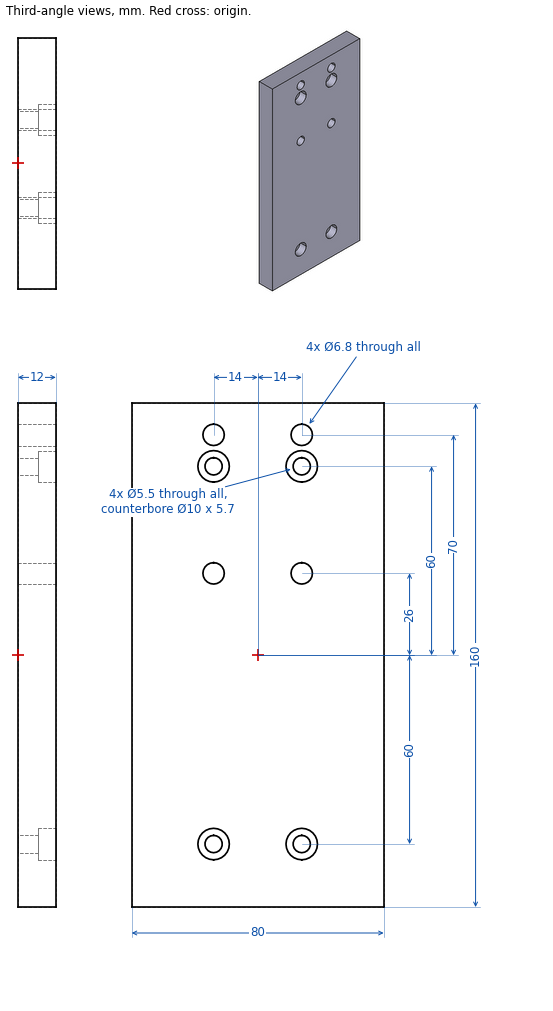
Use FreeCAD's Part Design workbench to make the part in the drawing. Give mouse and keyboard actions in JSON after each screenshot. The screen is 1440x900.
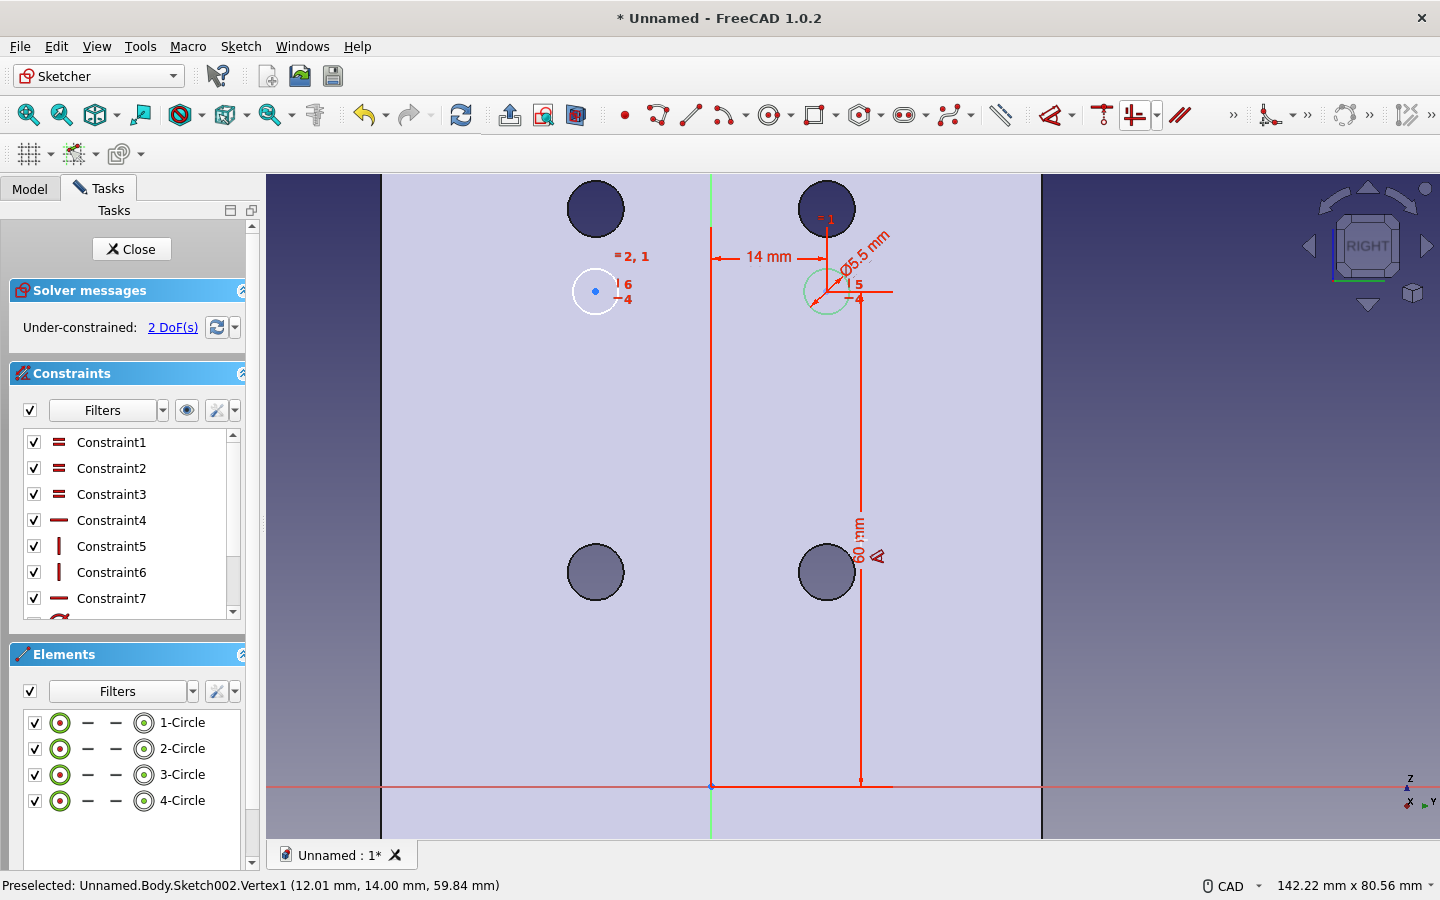
{"action": "left_click", "coordinate": [596, 292]}
{"action": "left_click", "coordinate": [654, 258]}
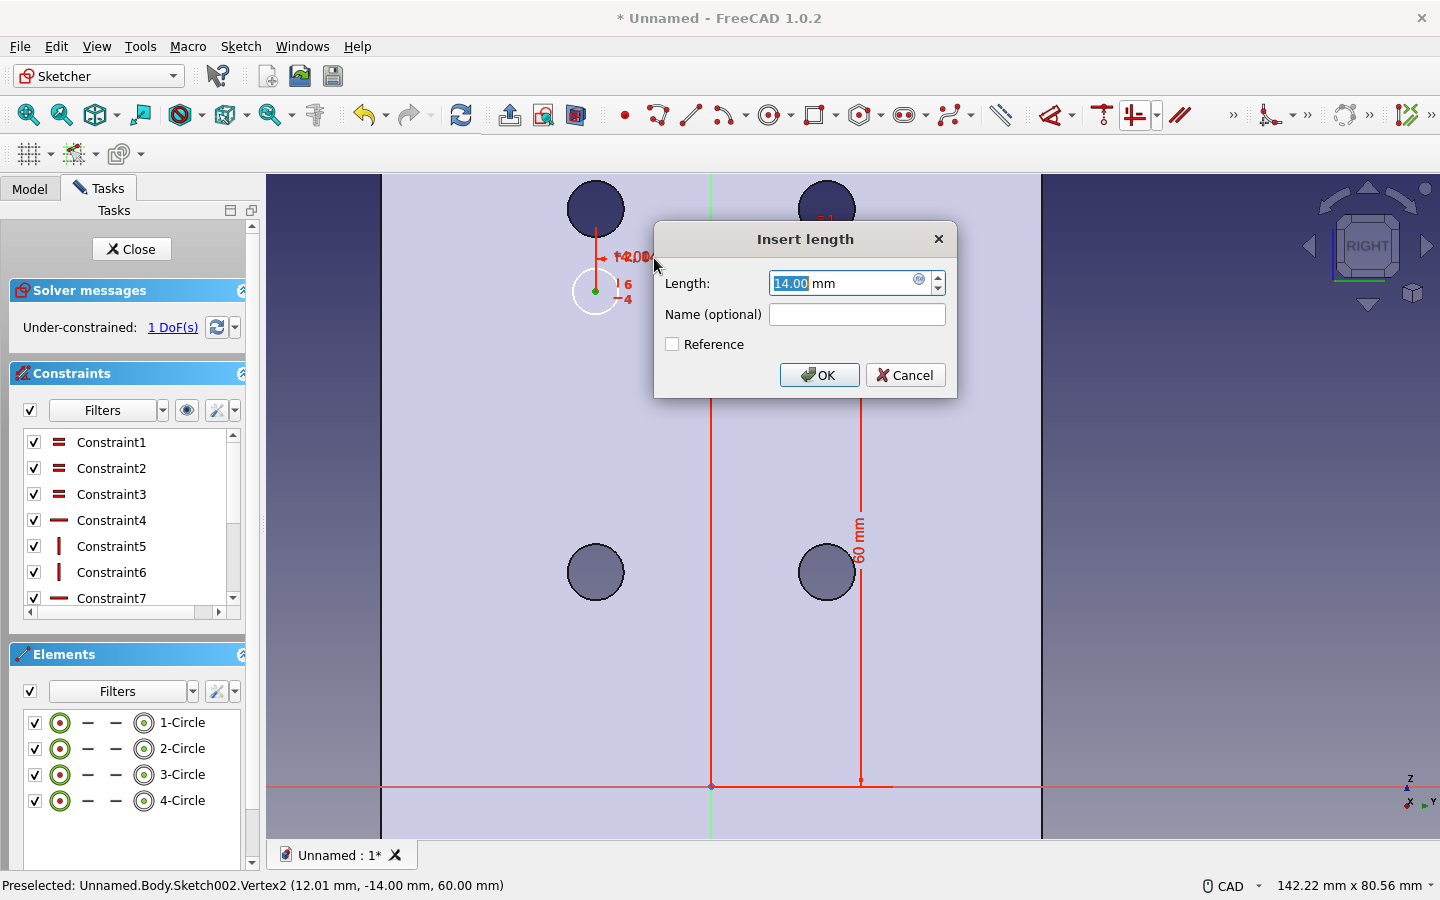
{"action": "type", "text": "14"}
{"action": "key", "text": "Return"}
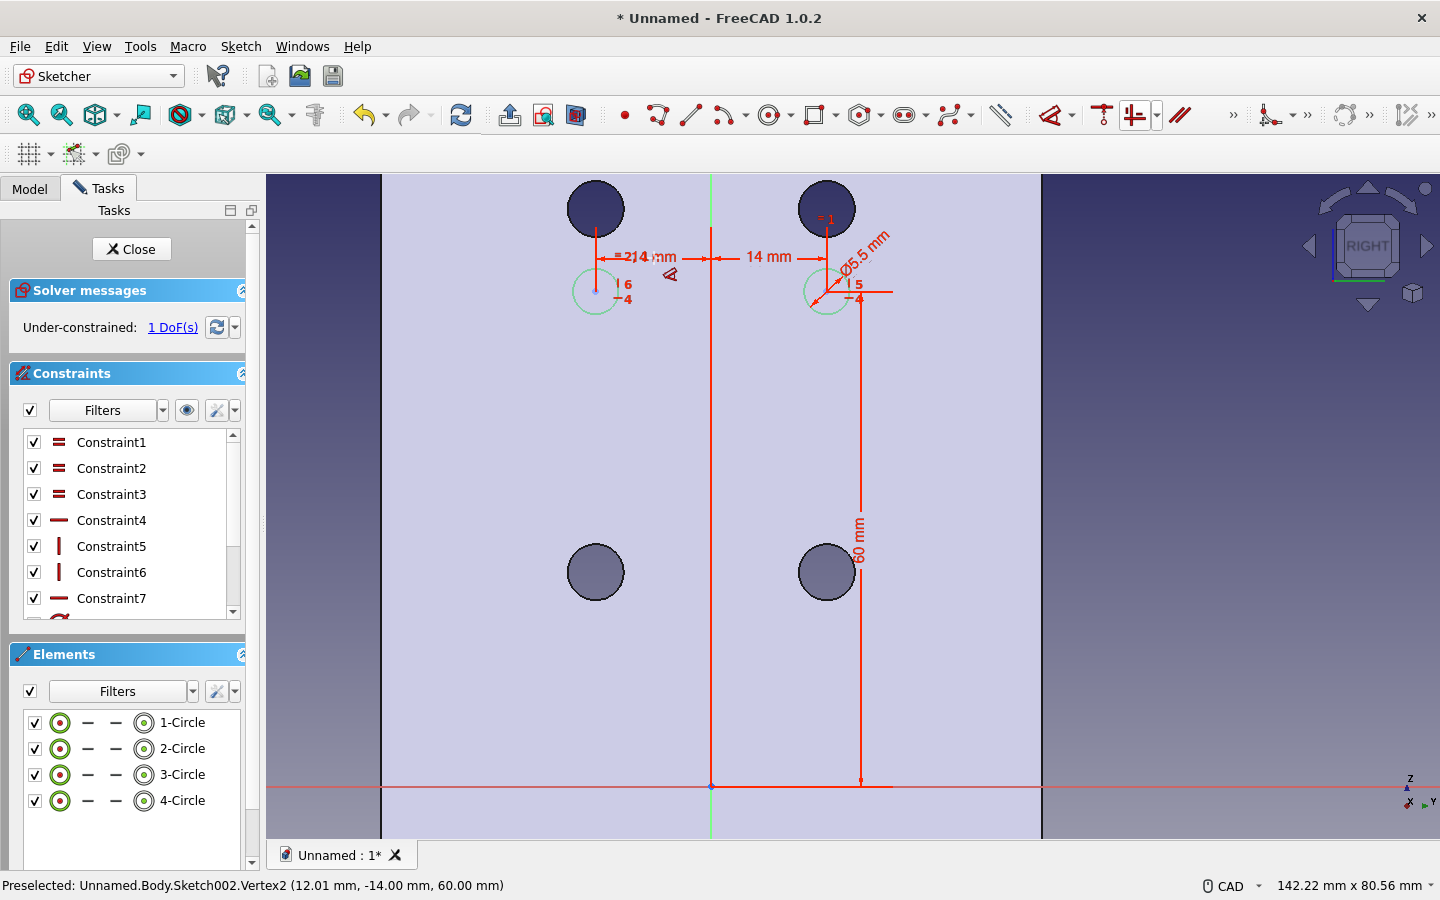
{"action": "scroll", "coordinate": [844, 278], "scroll_direction": "down", "scroll_amount": 4}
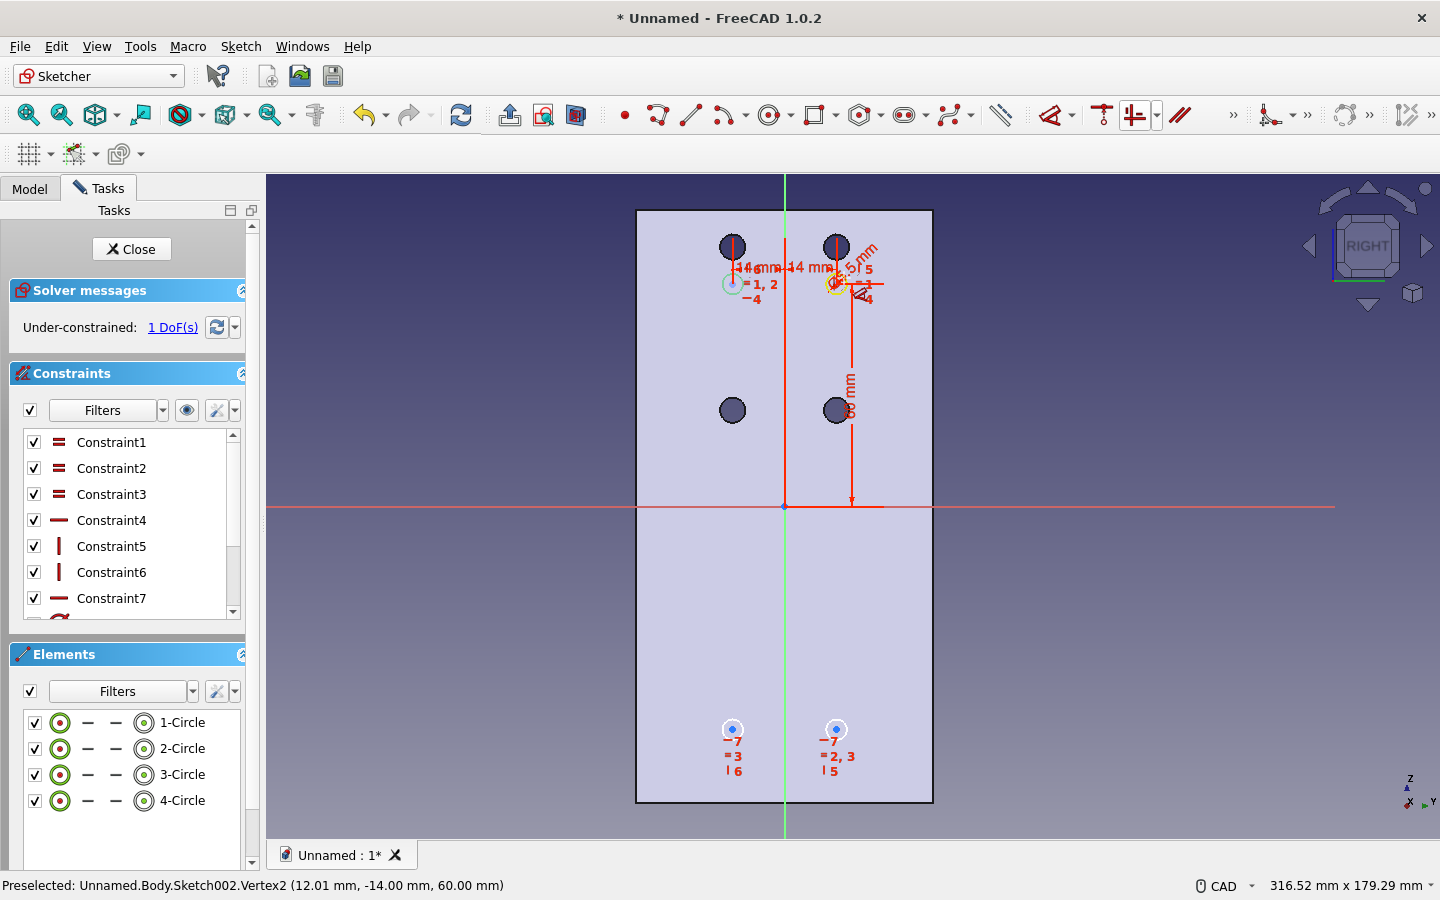
{"action": "left_click", "coordinate": [837, 730]}
{"action": "left_click", "coordinate": [871, 618]}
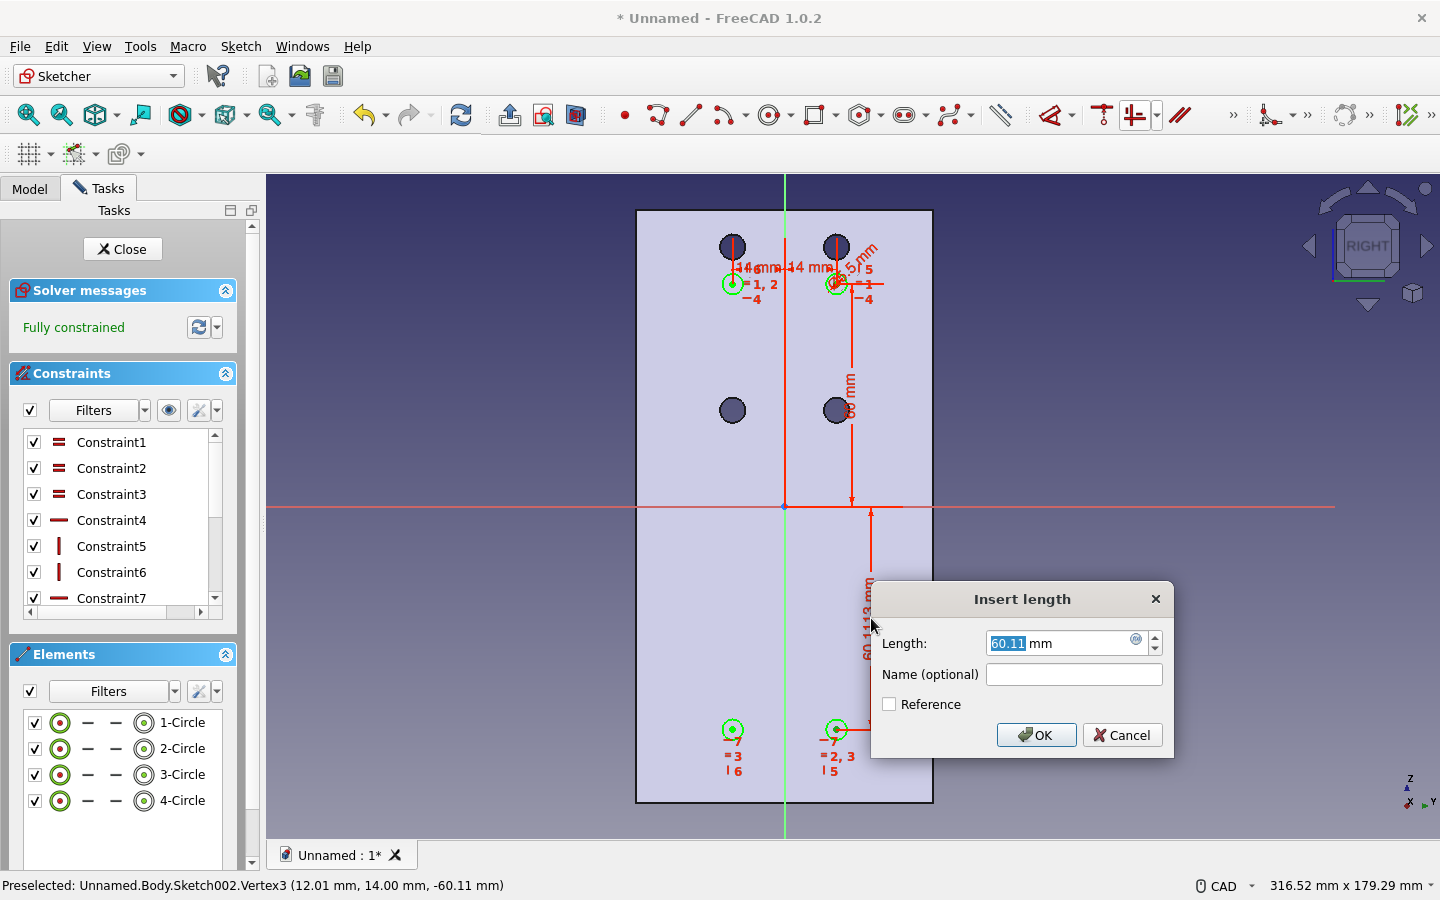
{"action": "type", "text": "60"}
{"action": "key", "text": "Return"}
{"action": "key", "text": "Escape"}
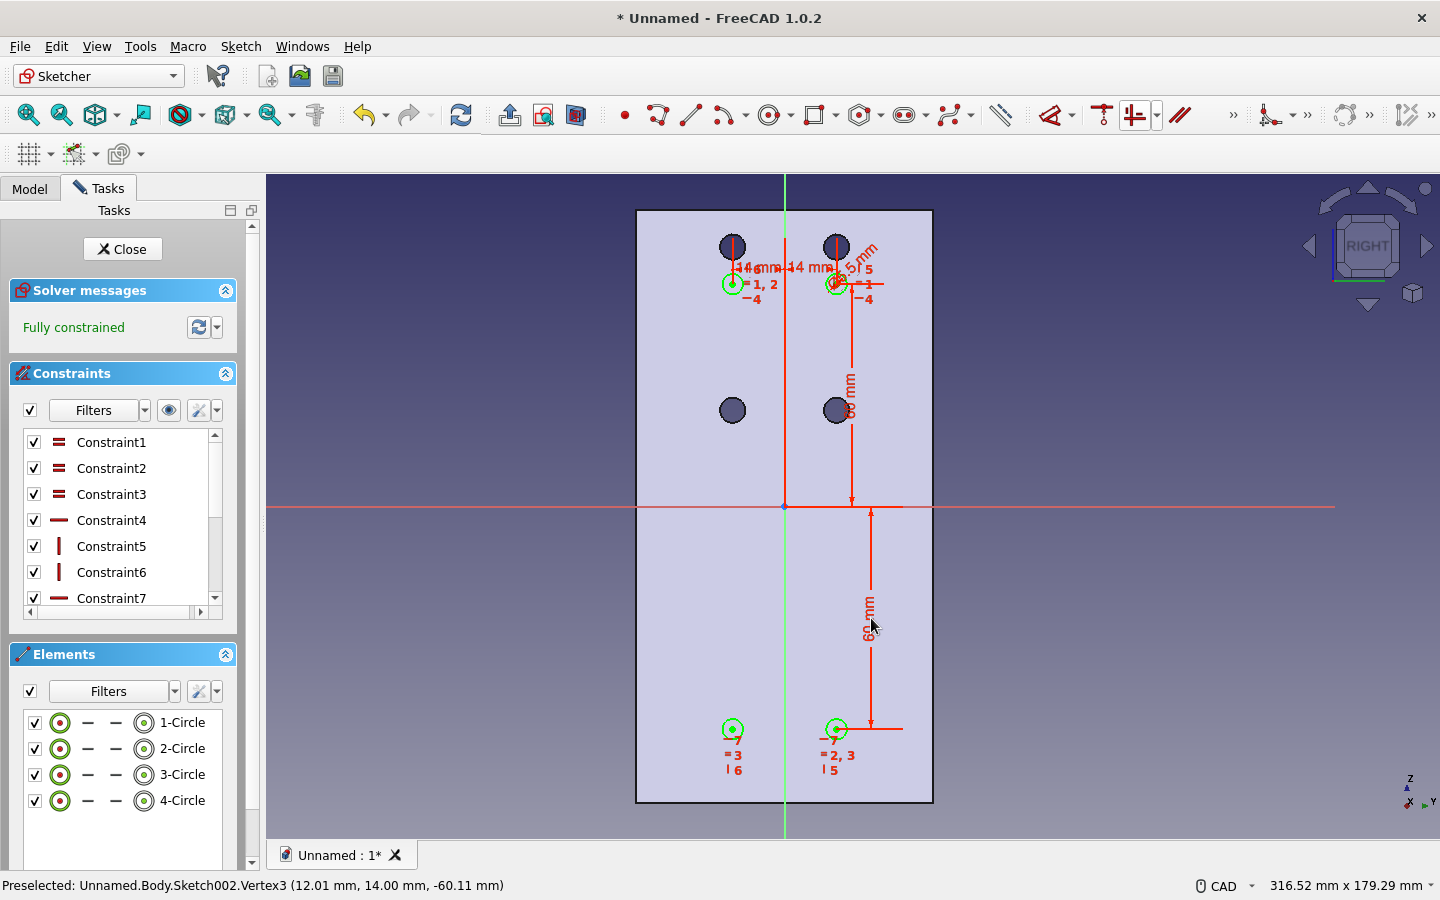
{"action": "left_click", "coordinate": [123, 249]}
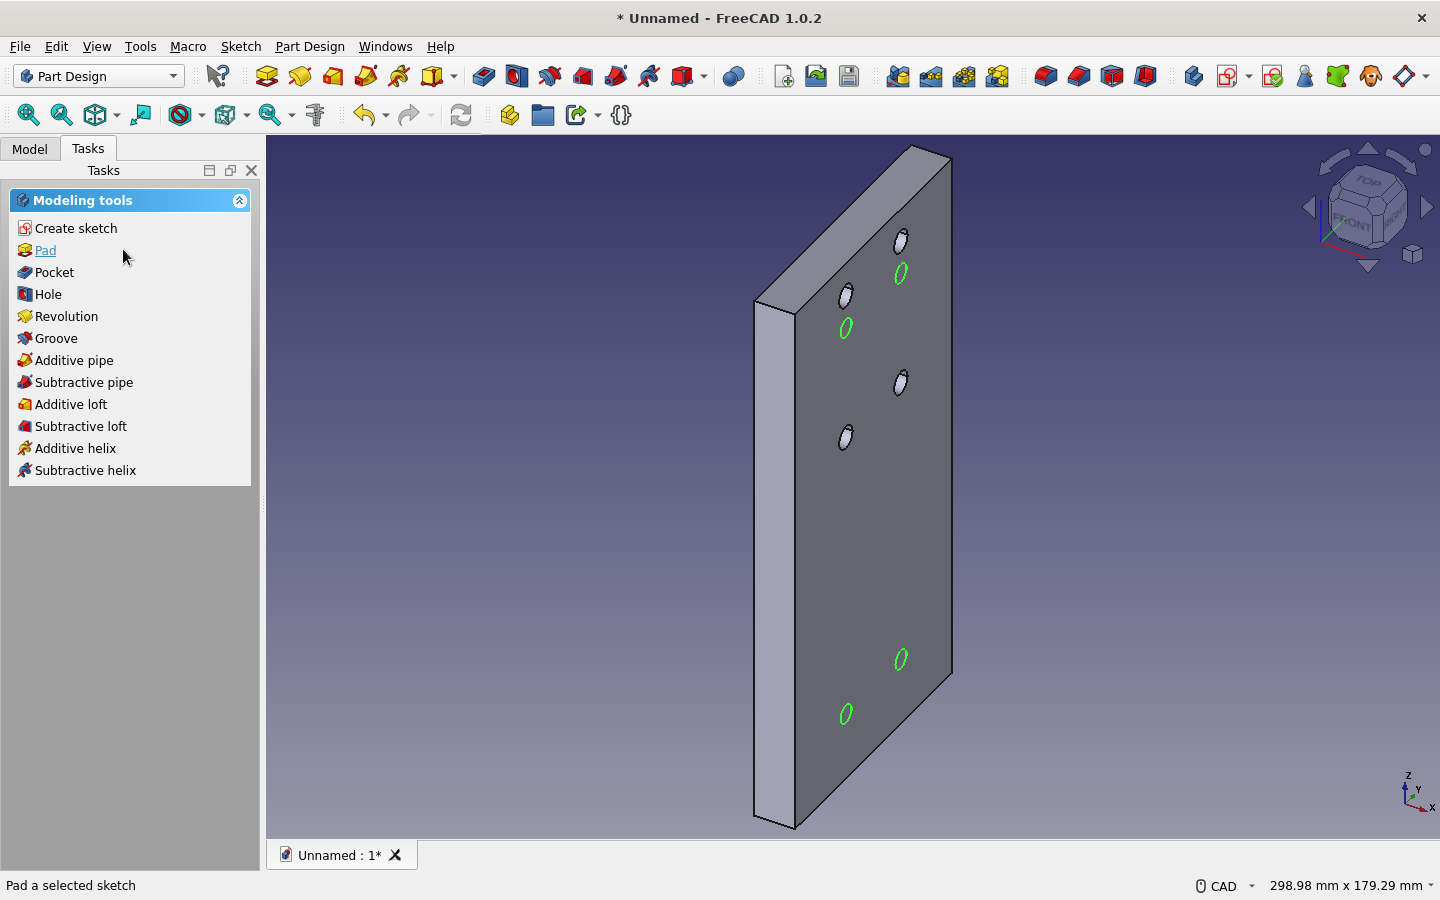
{"action": "left_click", "coordinate": [517, 76]}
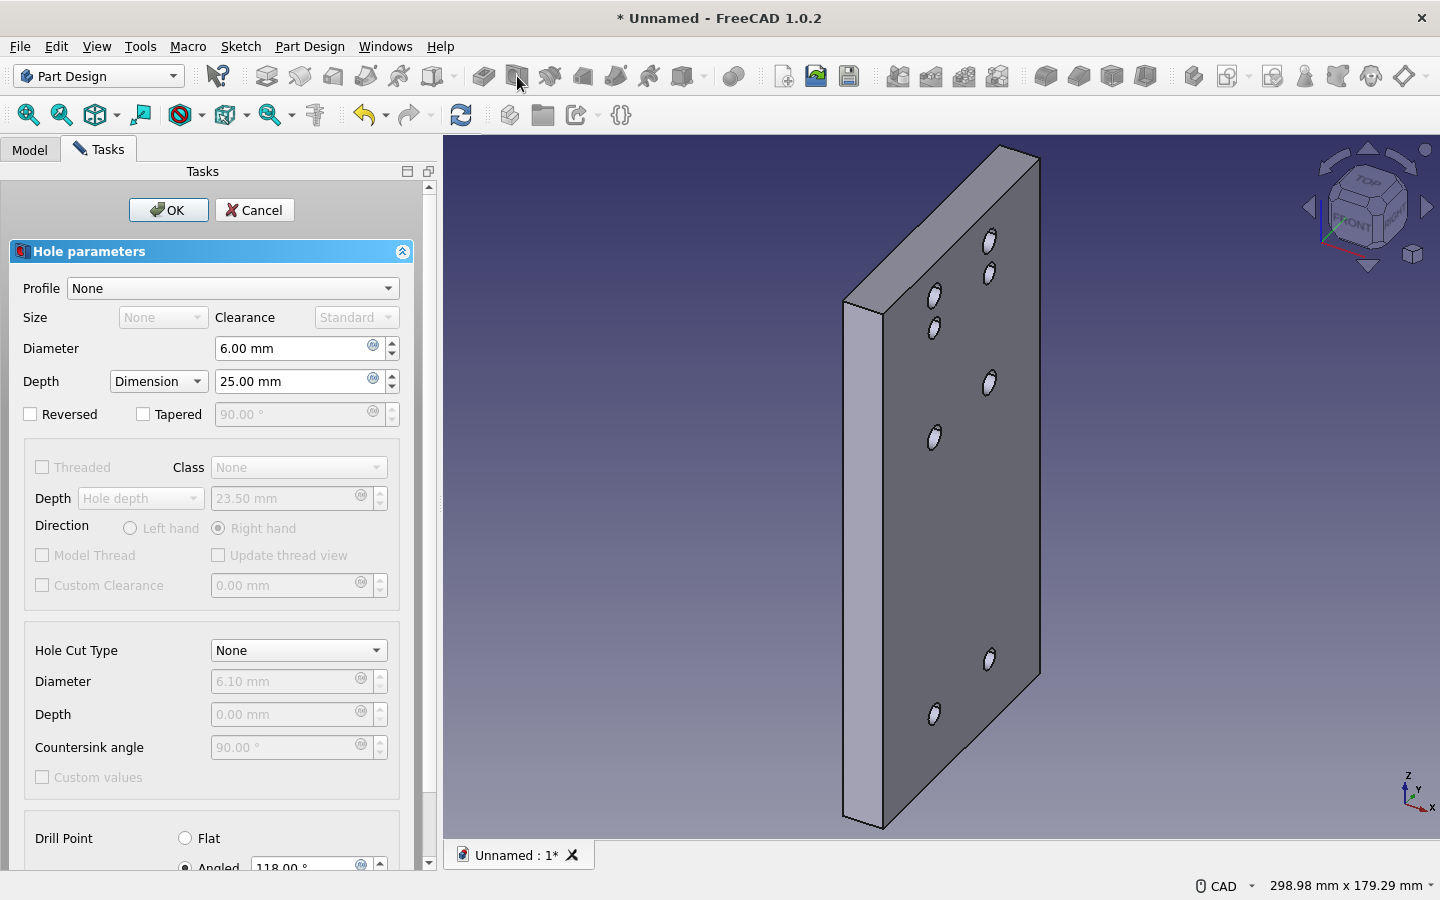
{"action": "triple_click", "coordinate": [300, 348]}